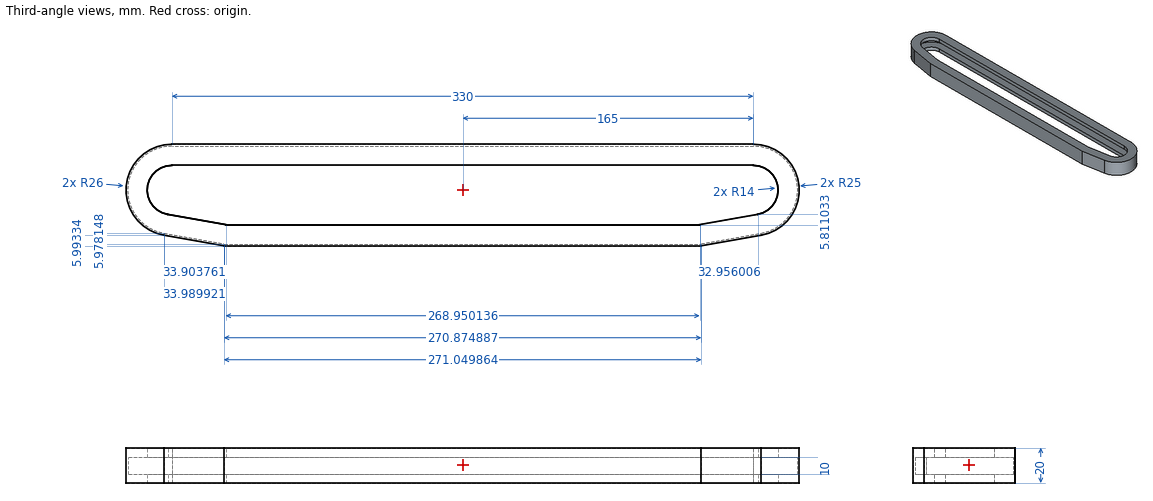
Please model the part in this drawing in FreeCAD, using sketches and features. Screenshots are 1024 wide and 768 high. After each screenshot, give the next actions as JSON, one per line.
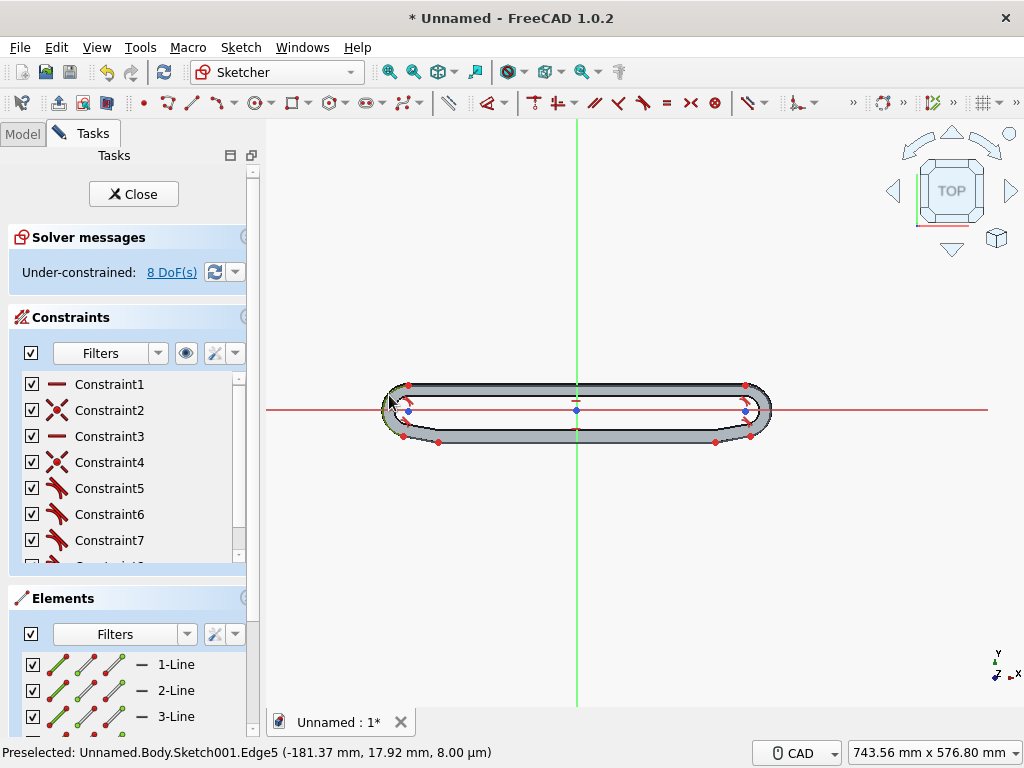
{"action": "left_click", "coordinate": [768, 423]}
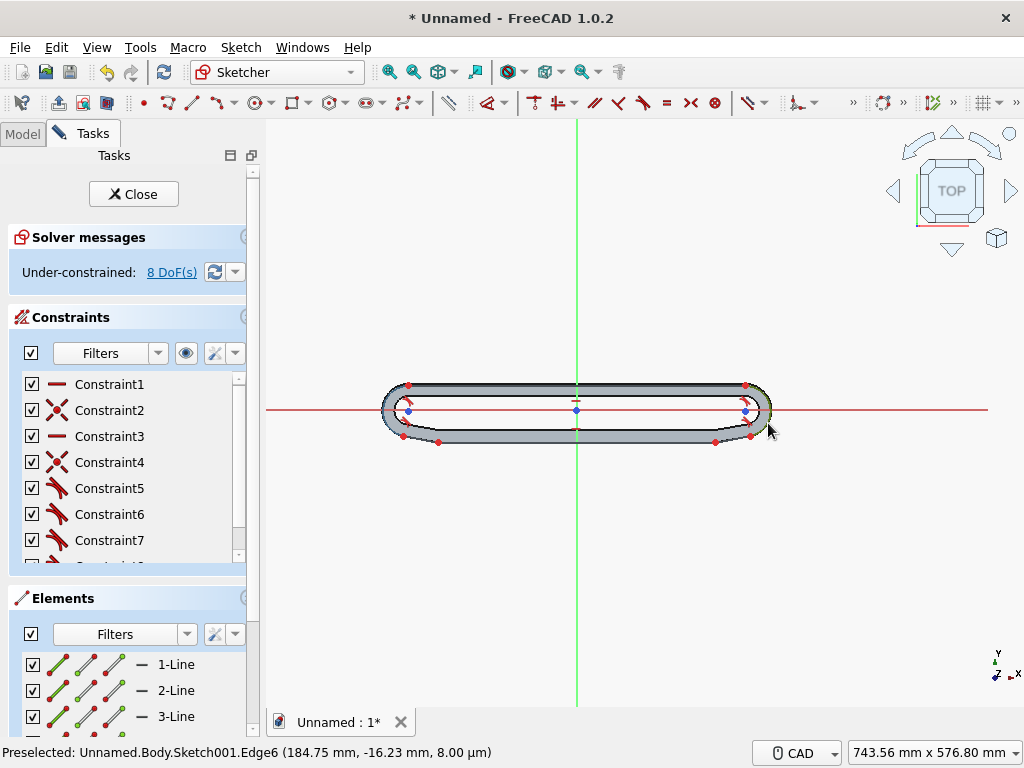
{"action": "left_click", "coordinate": [668, 104]}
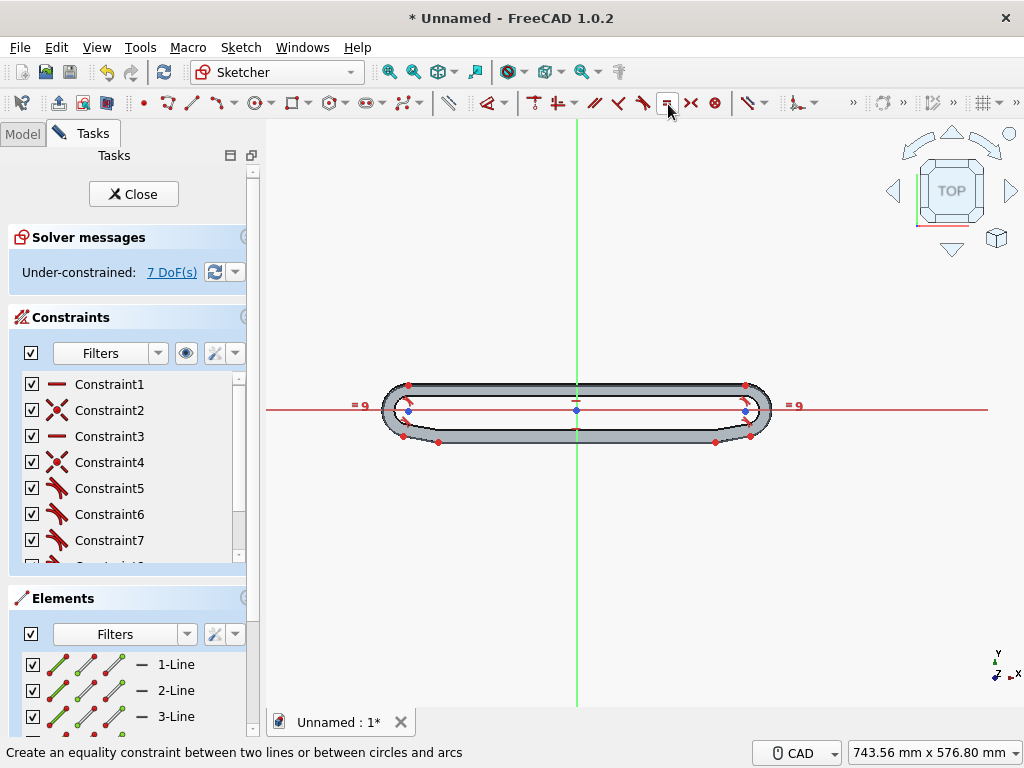
{"action": "left_click", "coordinate": [408, 411]}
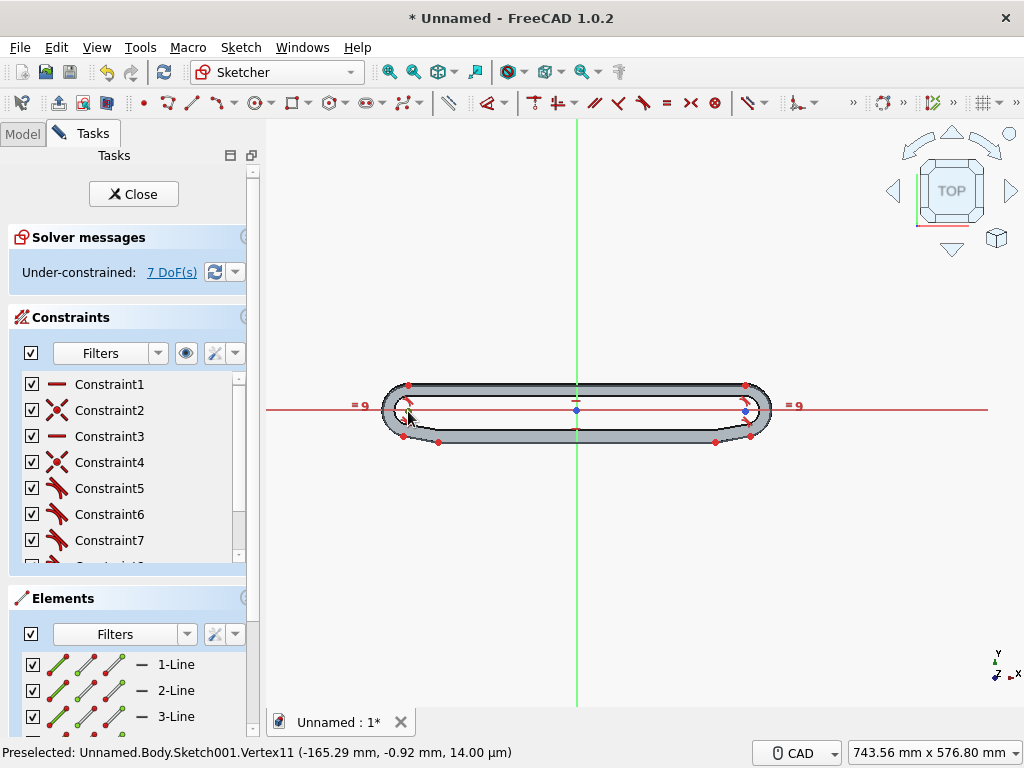
{"action": "left_click", "coordinate": [334, 410]}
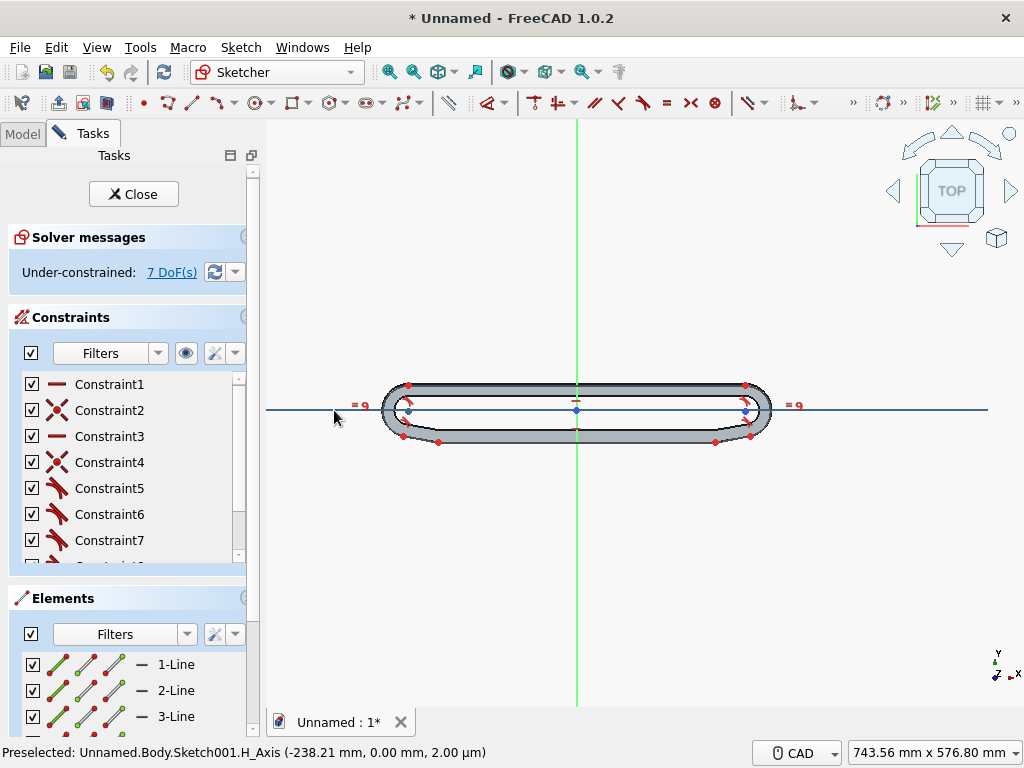
{"action": "left_click", "coordinate": [534, 104]}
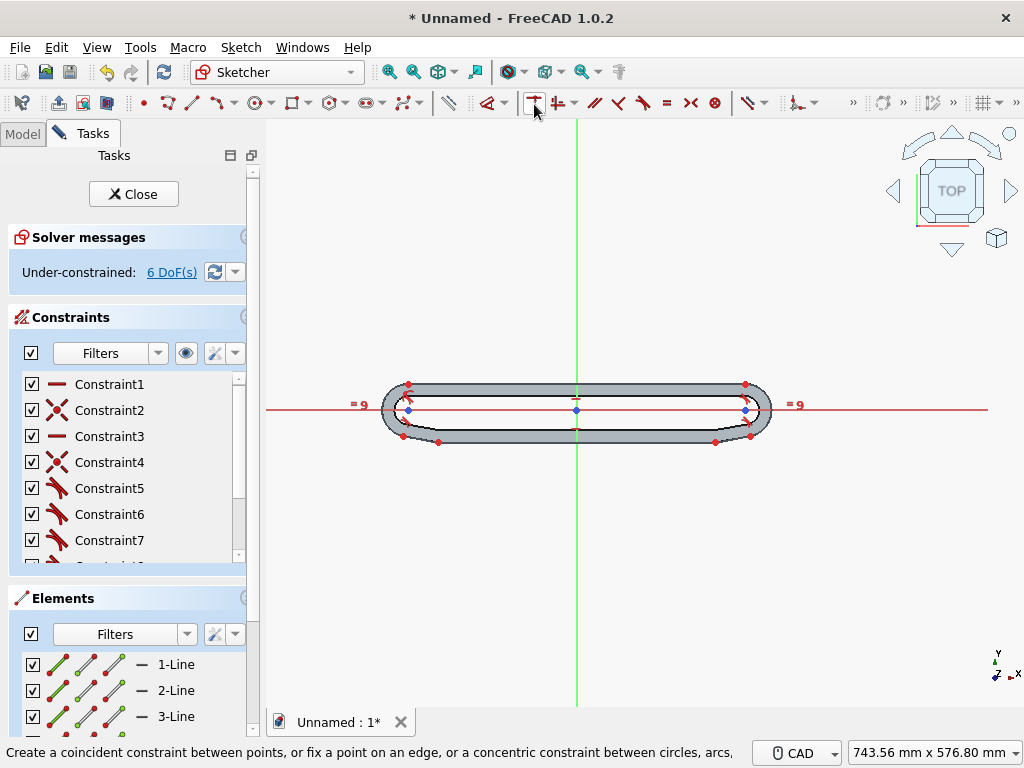
{"action": "left_click", "coordinate": [488, 104]}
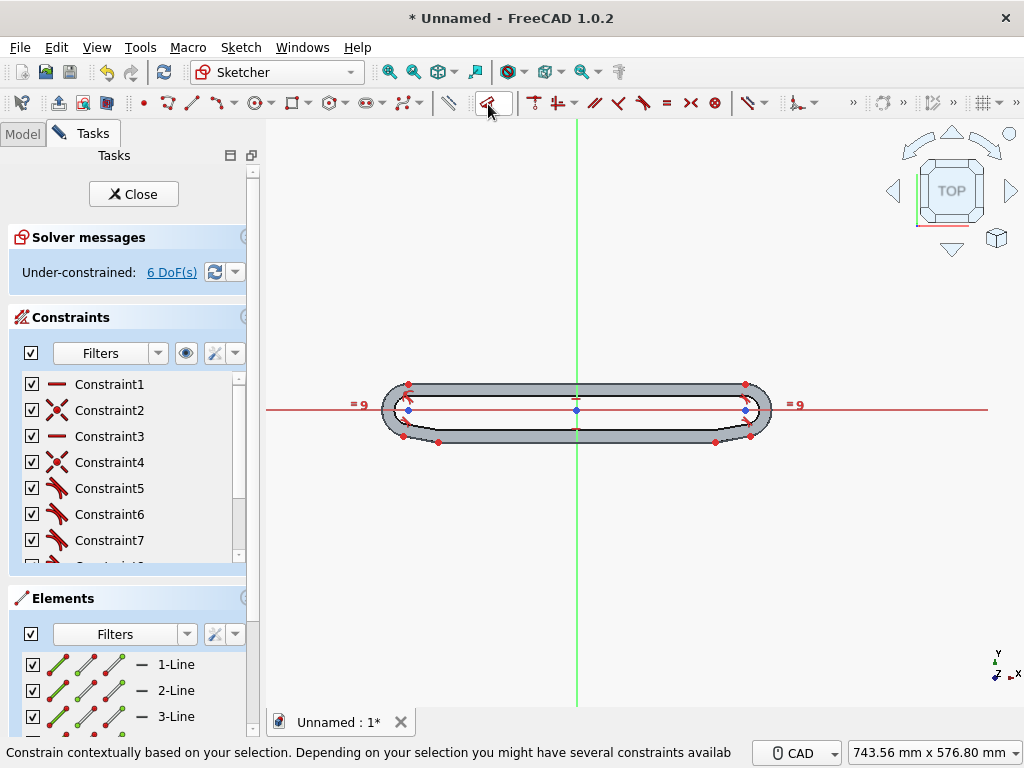
{"action": "scroll", "coordinate": [388, 394], "scroll_direction": "up", "scroll_amount": 3}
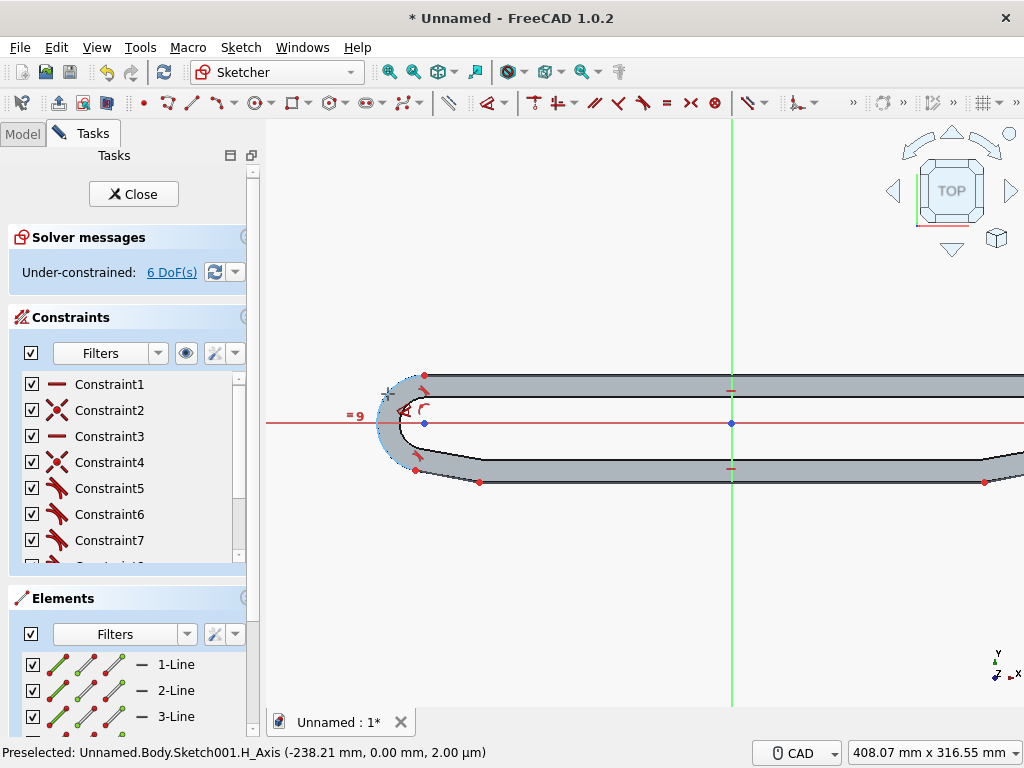
{"action": "left_click", "coordinate": [388, 393]}
{"action": "left_click", "coordinate": [363, 373]}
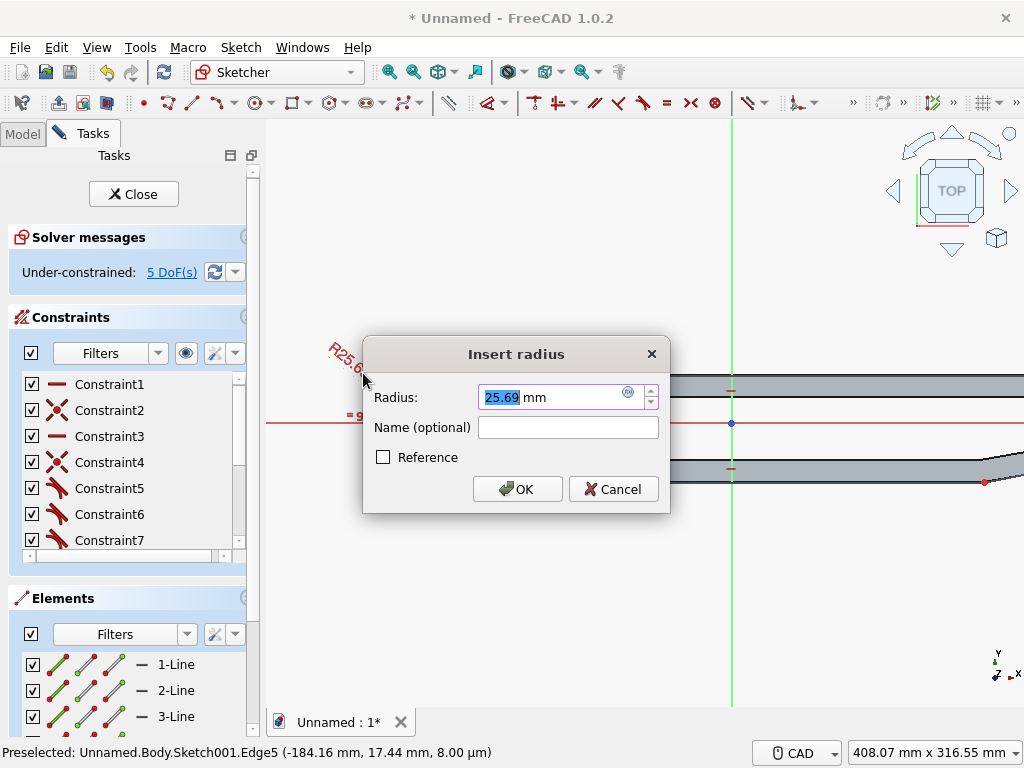
{"action": "type", "text": "25"}
{"action": "key", "text": "Return"}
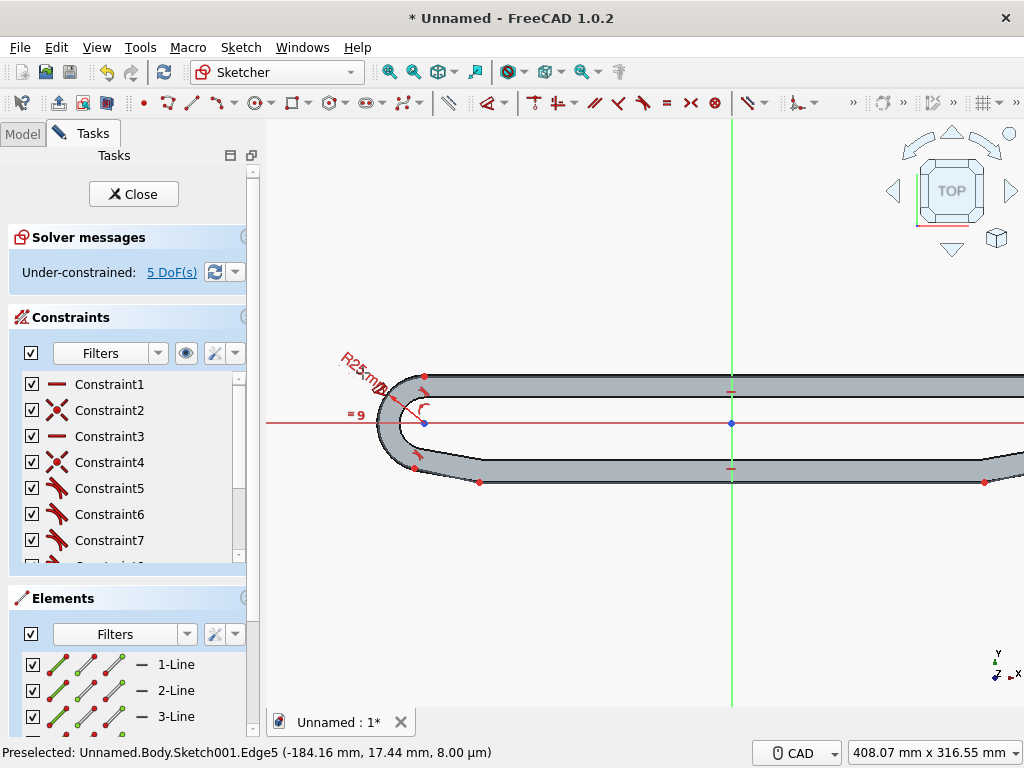
{"action": "left_click", "coordinate": [855, 377]}
{"action": "left_click", "coordinate": [642, 343]}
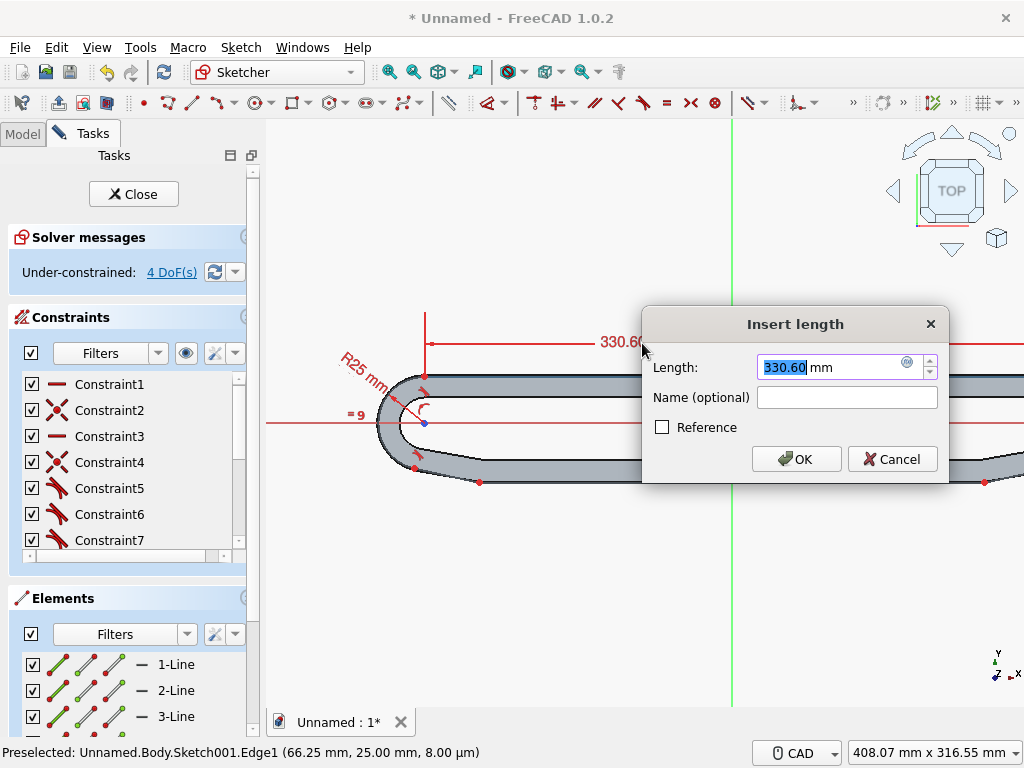
{"action": "type", "text": "330"}
{"action": "key", "text": "Return"}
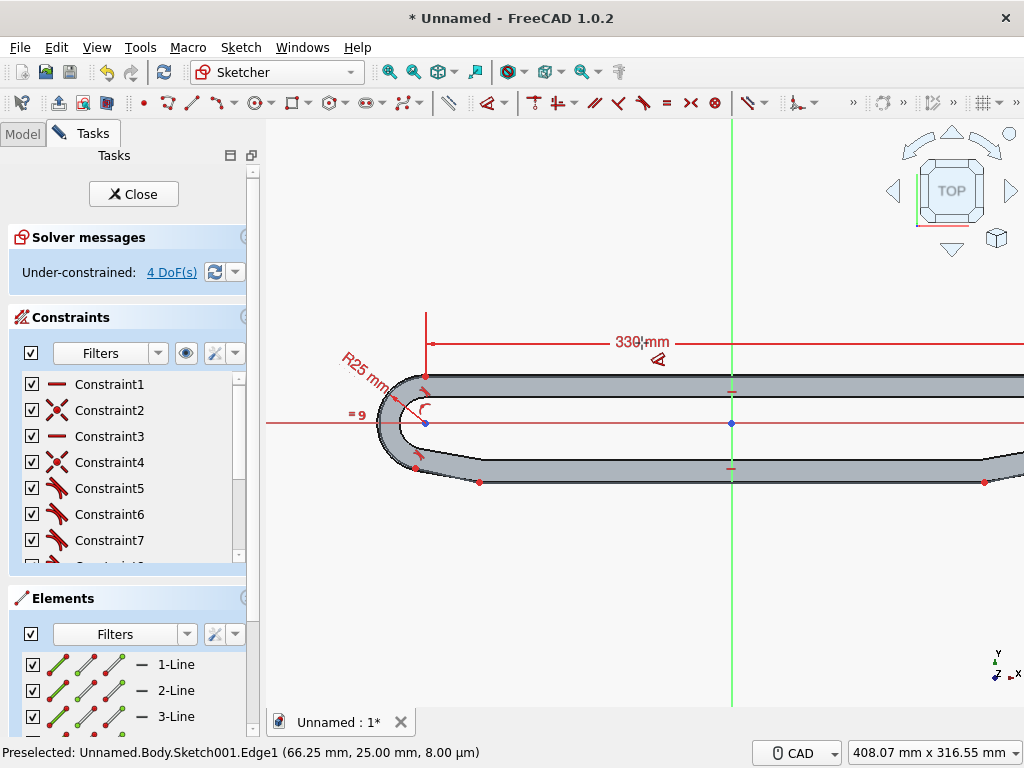
{"action": "scroll", "coordinate": [387, 394], "scroll_direction": "down", "scroll_amount": 3}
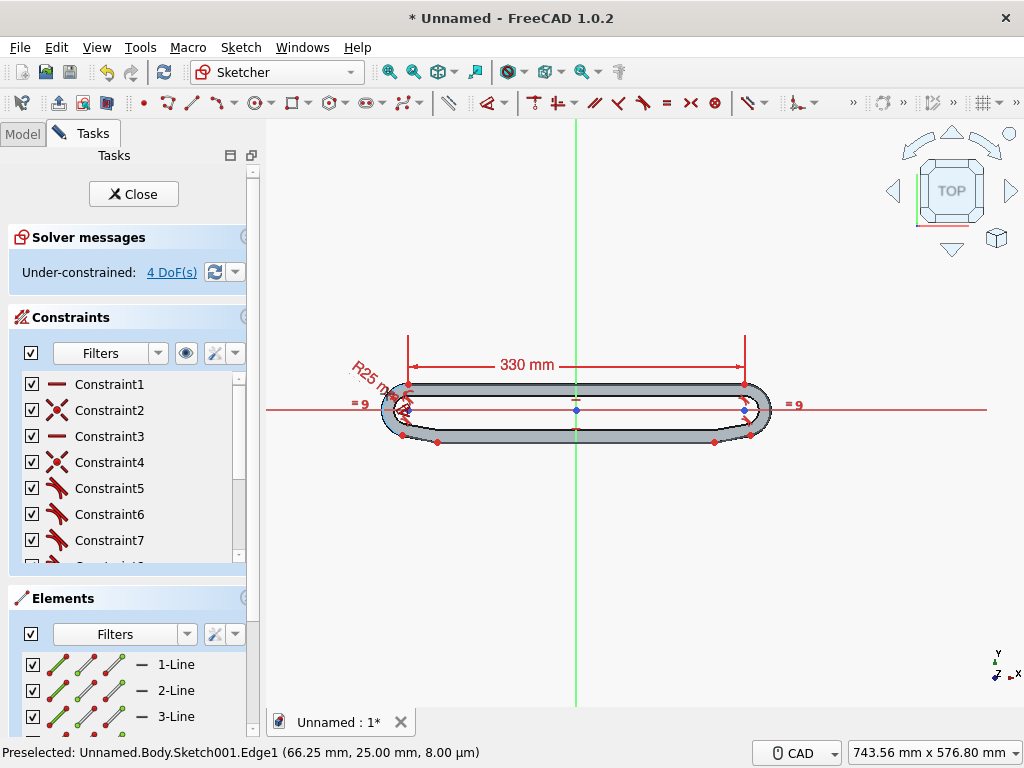
{"action": "left_click", "coordinate": [745, 385]}
{"action": "left_click", "coordinate": [661, 351]}